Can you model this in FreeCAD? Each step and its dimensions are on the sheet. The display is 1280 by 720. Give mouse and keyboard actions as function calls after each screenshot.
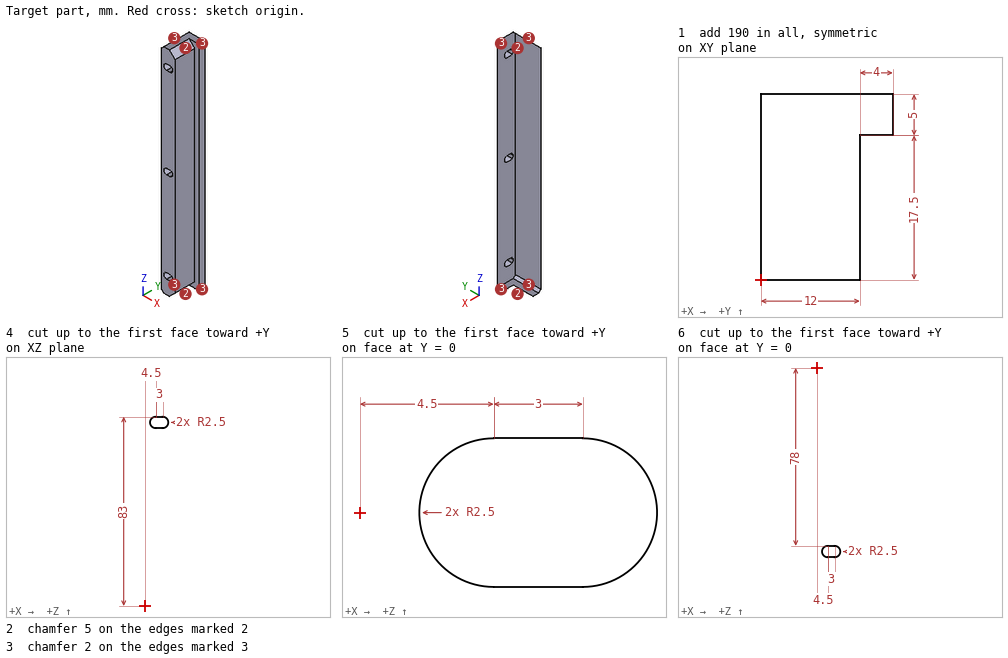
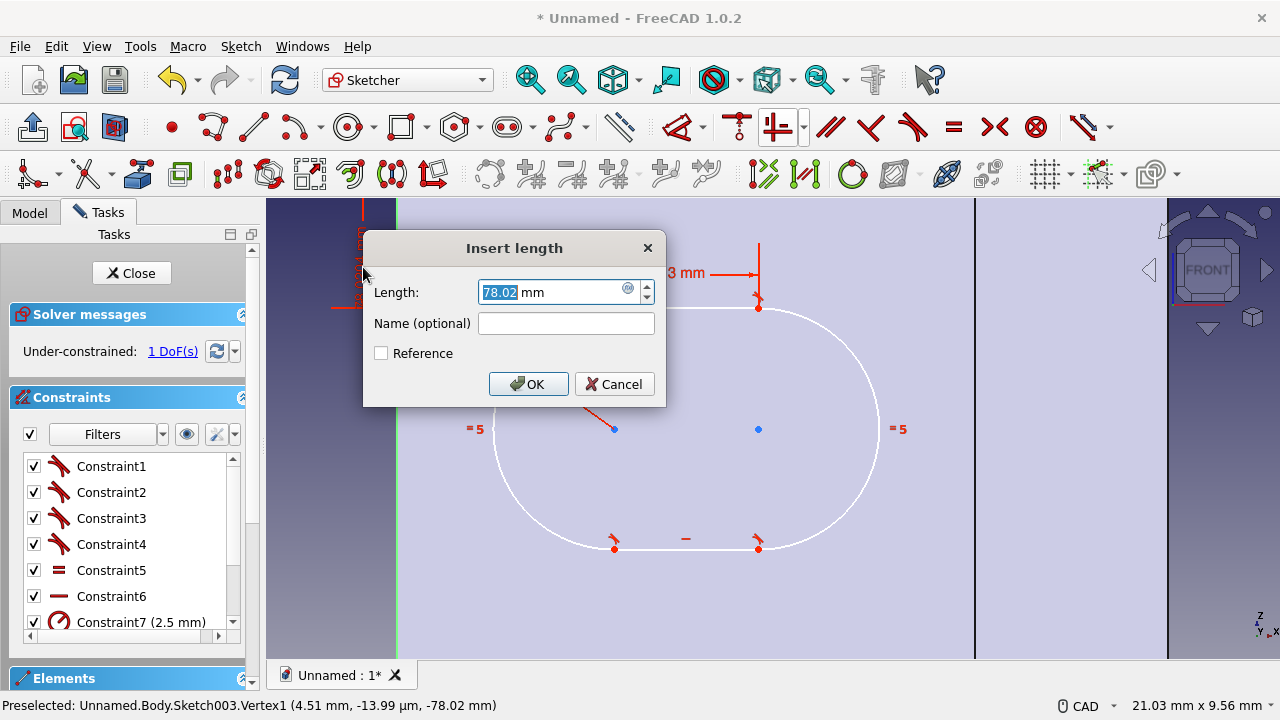
text(78)
key(Return)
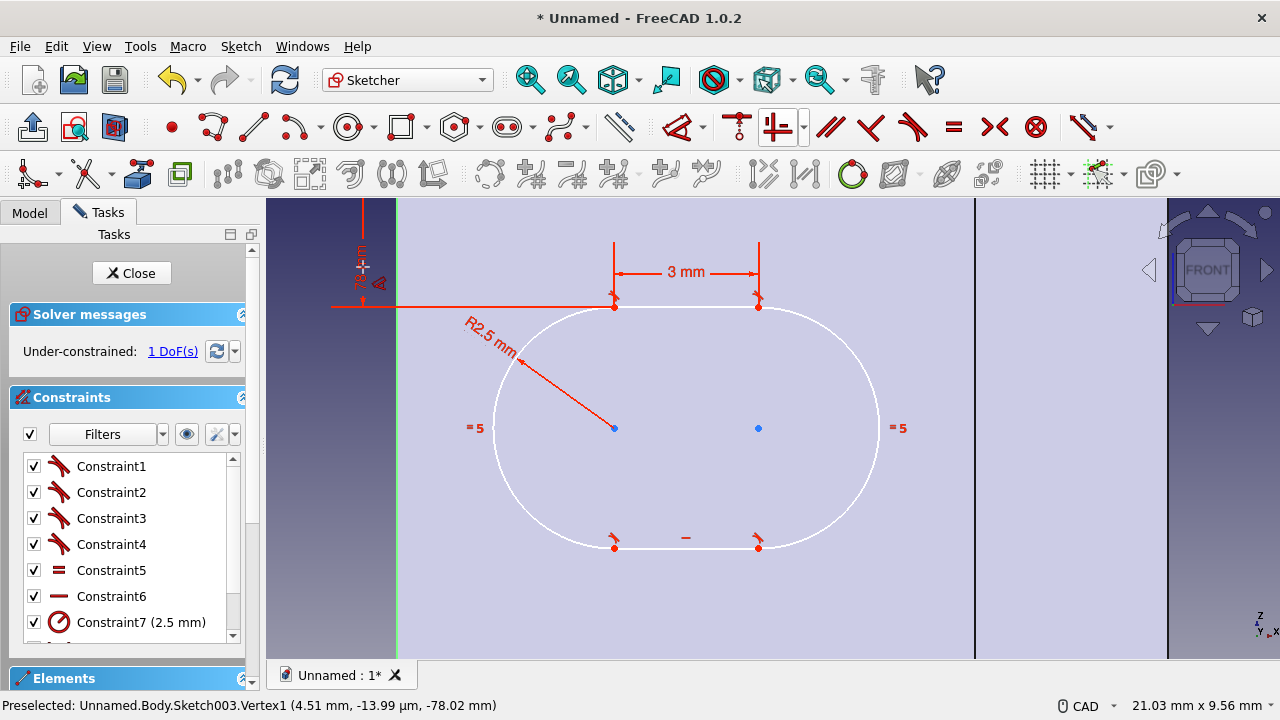
click(614, 307)
click(581, 341)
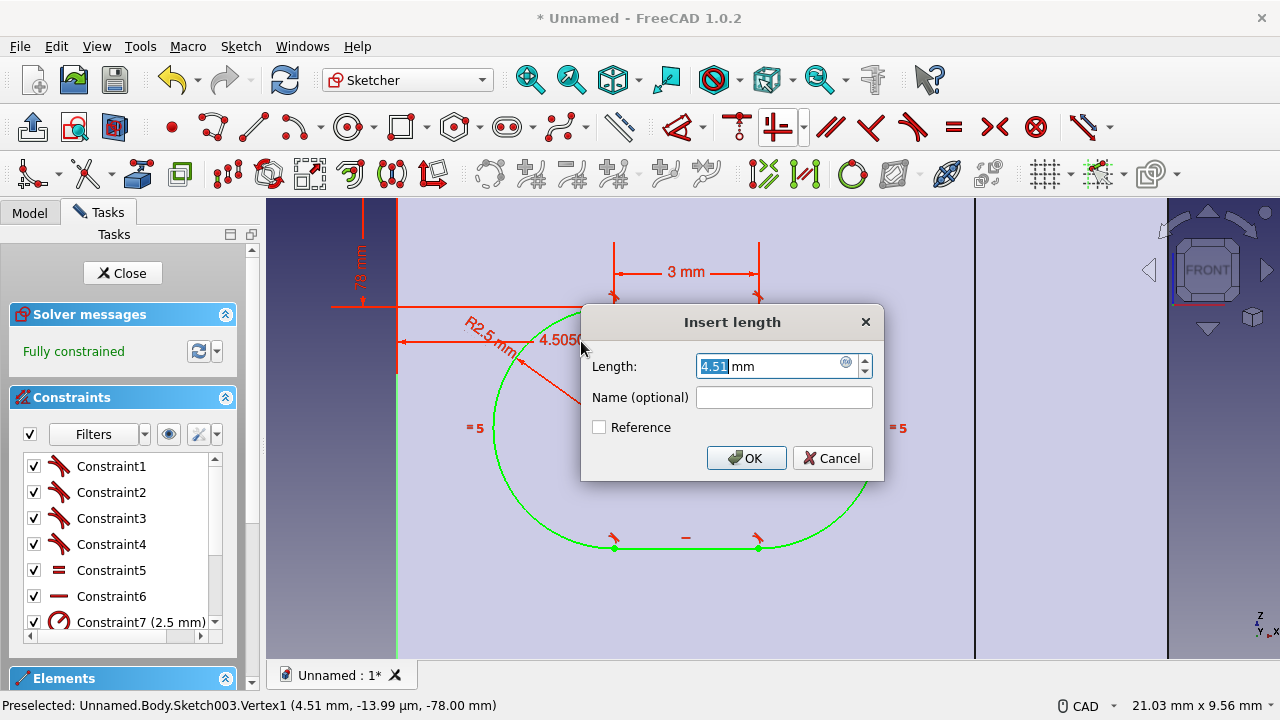
text(4.5)
key(Return)
key(Escape)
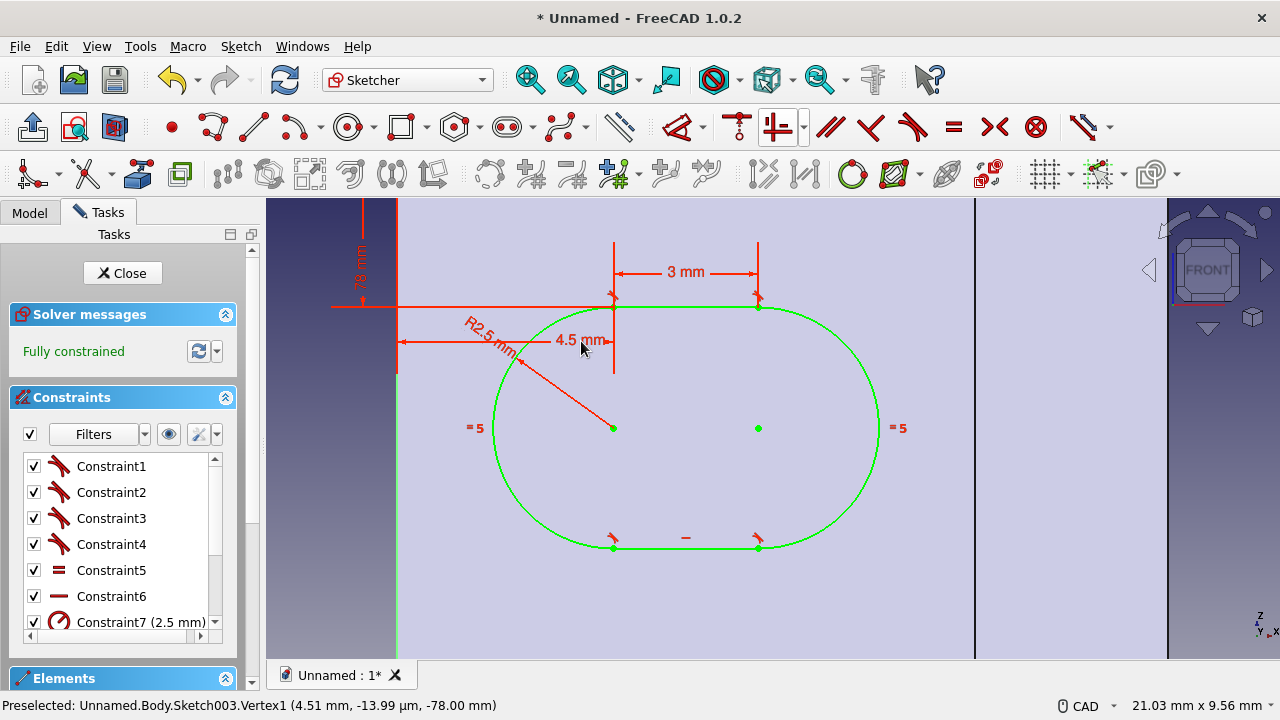
click(123, 273)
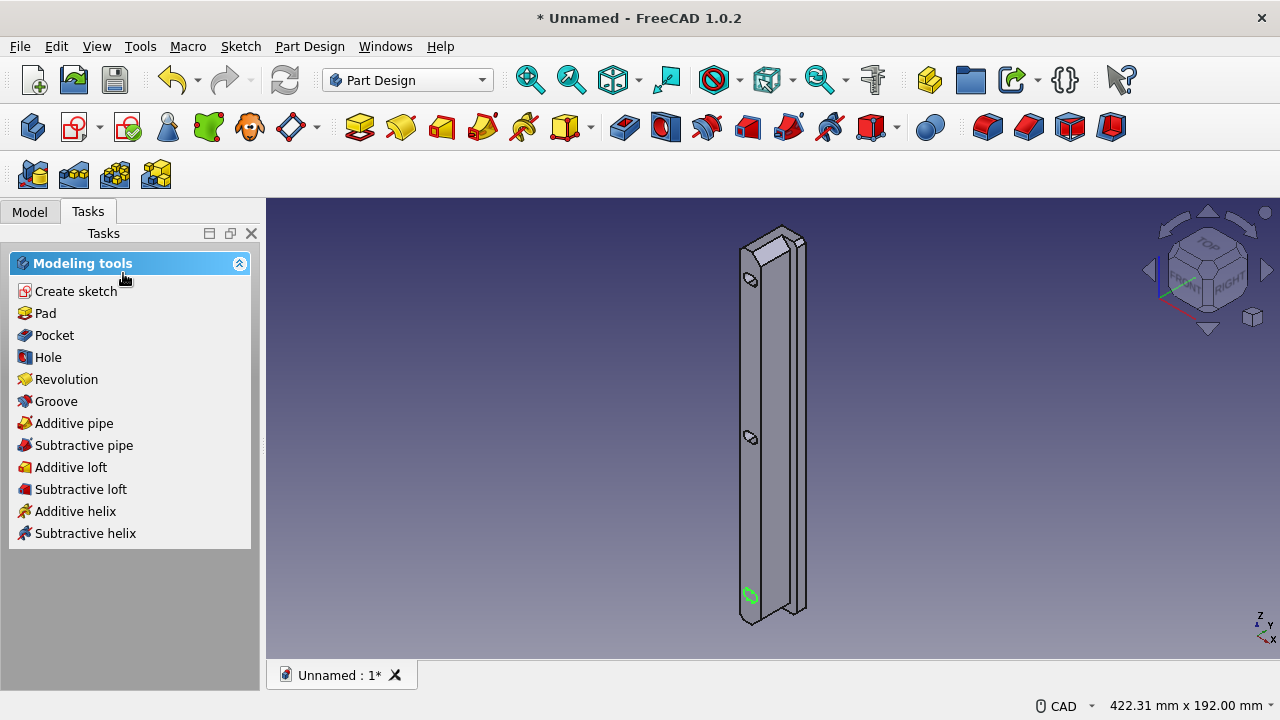
click(625, 128)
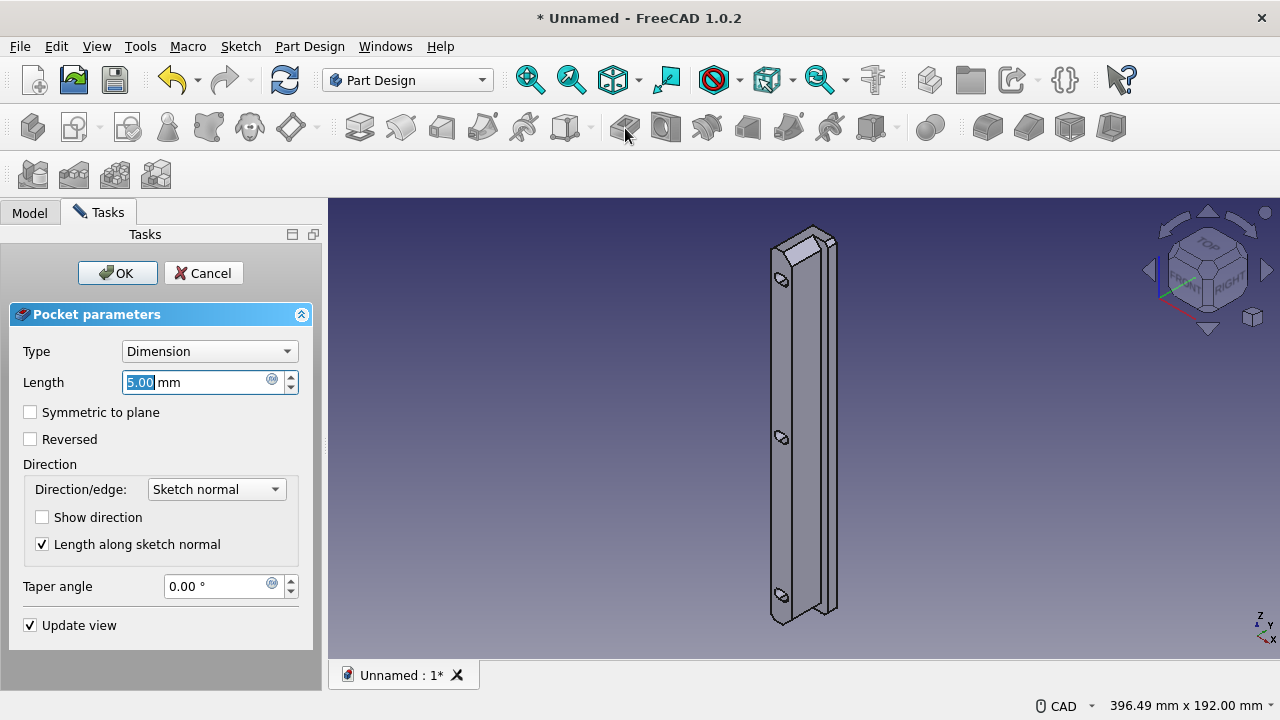
click(210, 352)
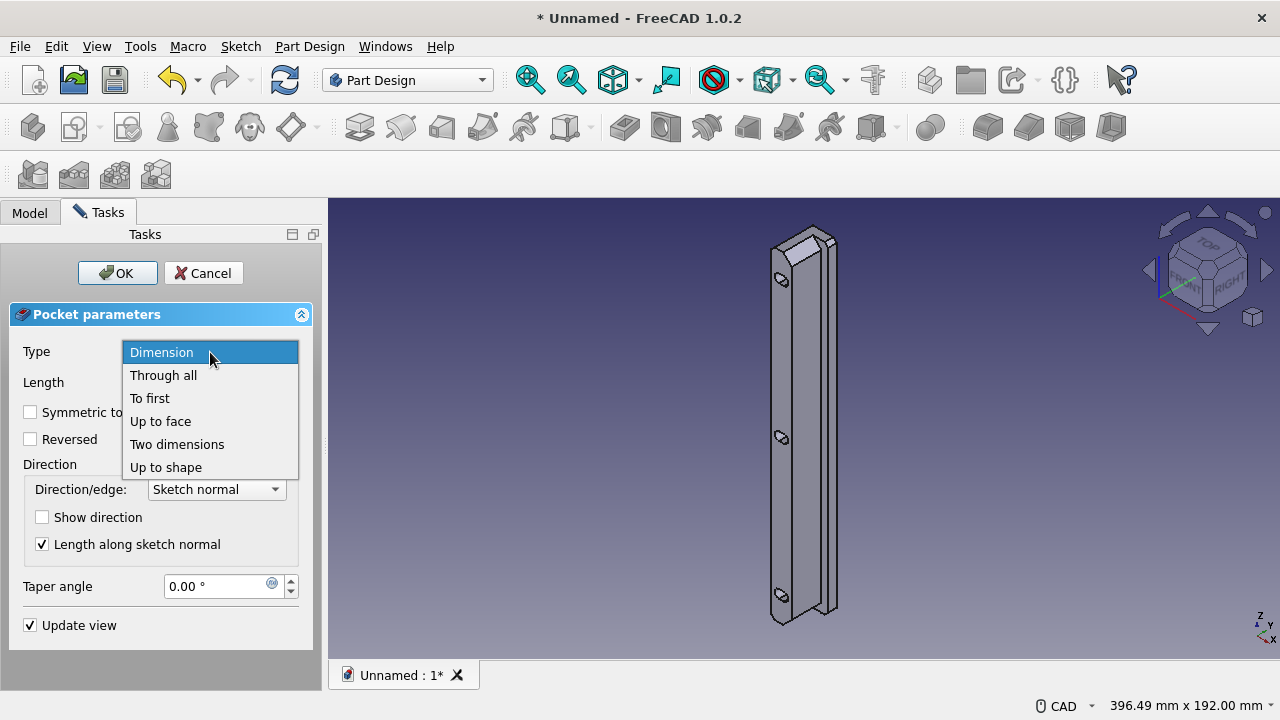
click(208, 398)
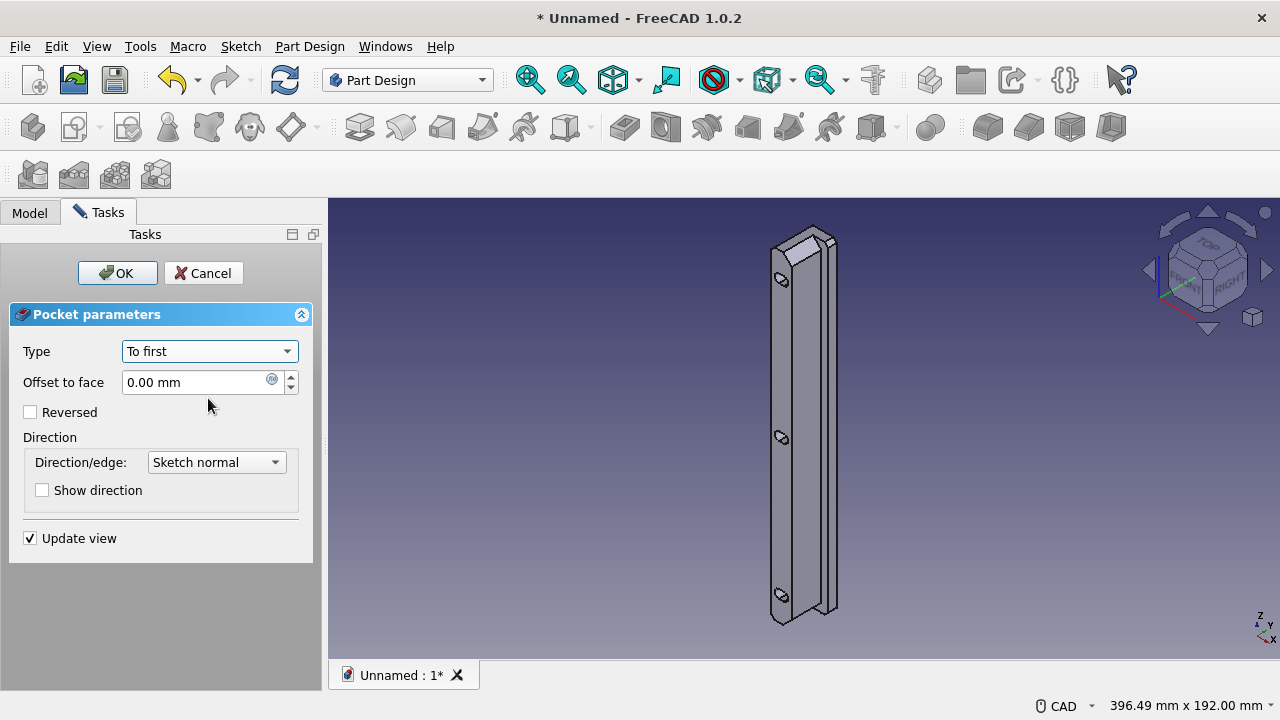
click(118, 273)